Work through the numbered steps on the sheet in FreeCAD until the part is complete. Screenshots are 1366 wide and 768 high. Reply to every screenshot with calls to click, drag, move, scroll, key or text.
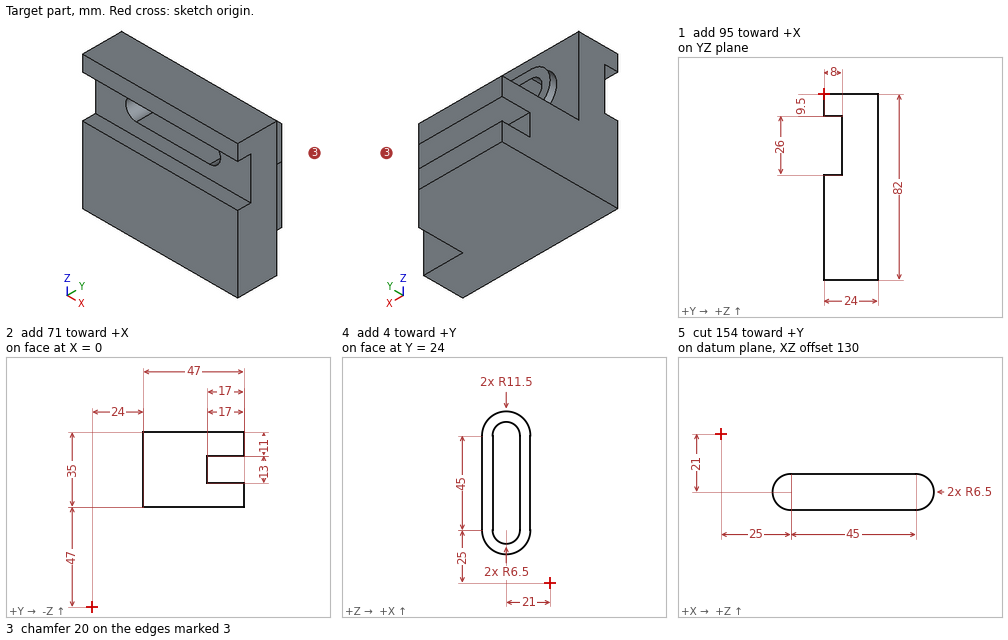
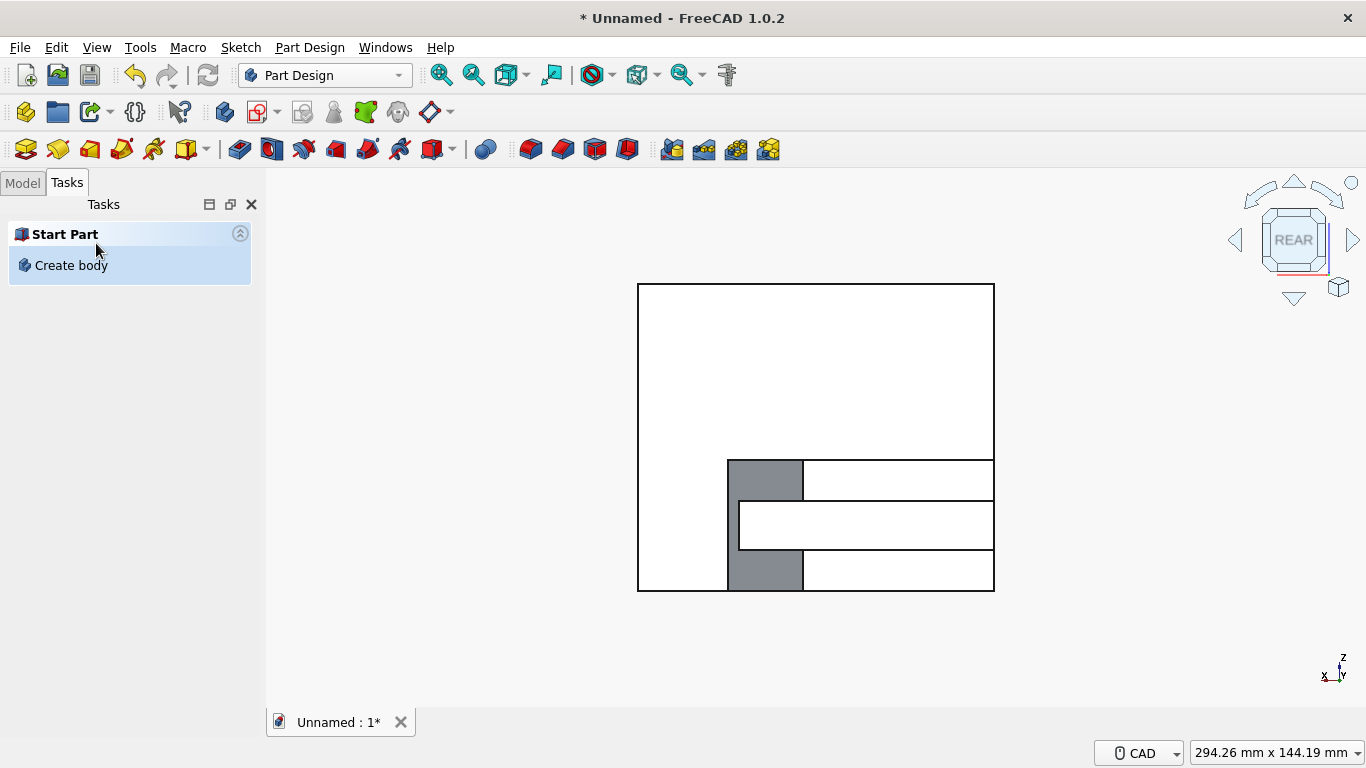
click(715, 393)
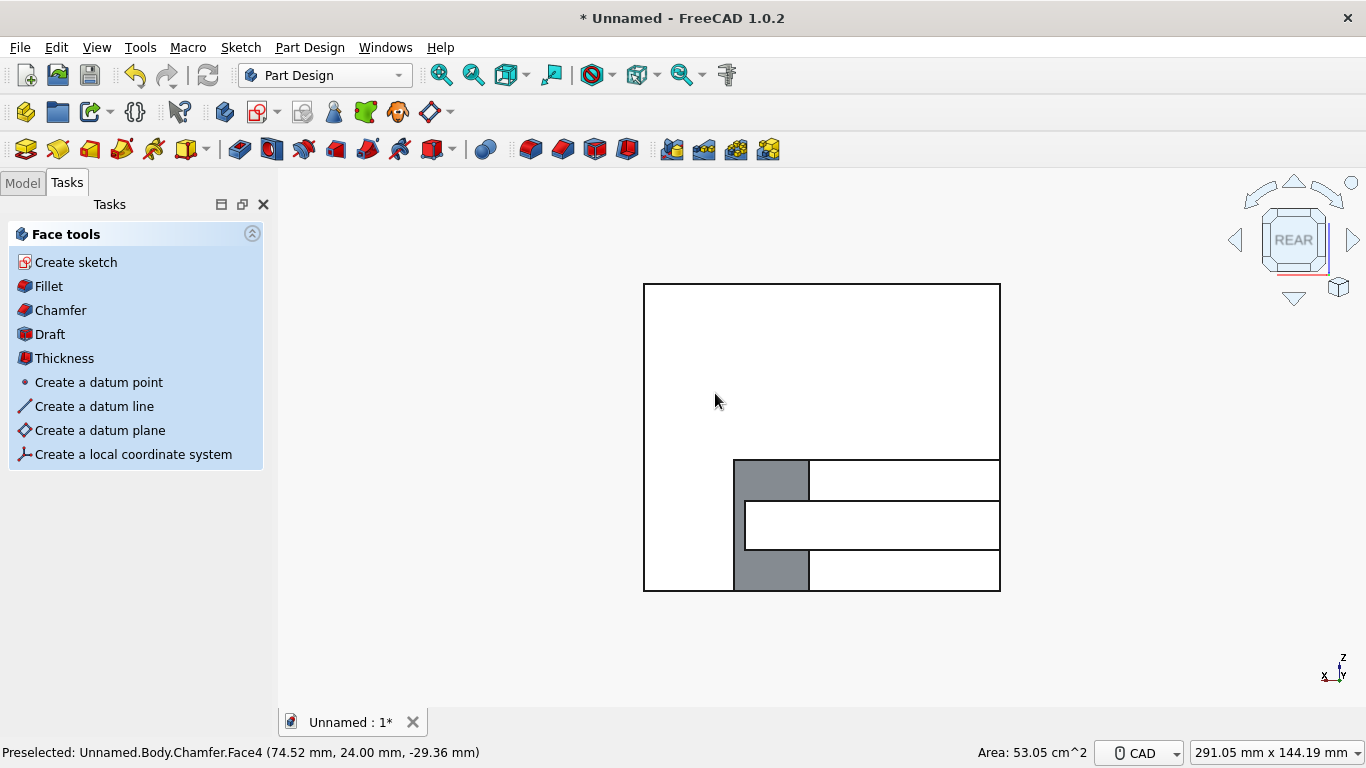
click(258, 112)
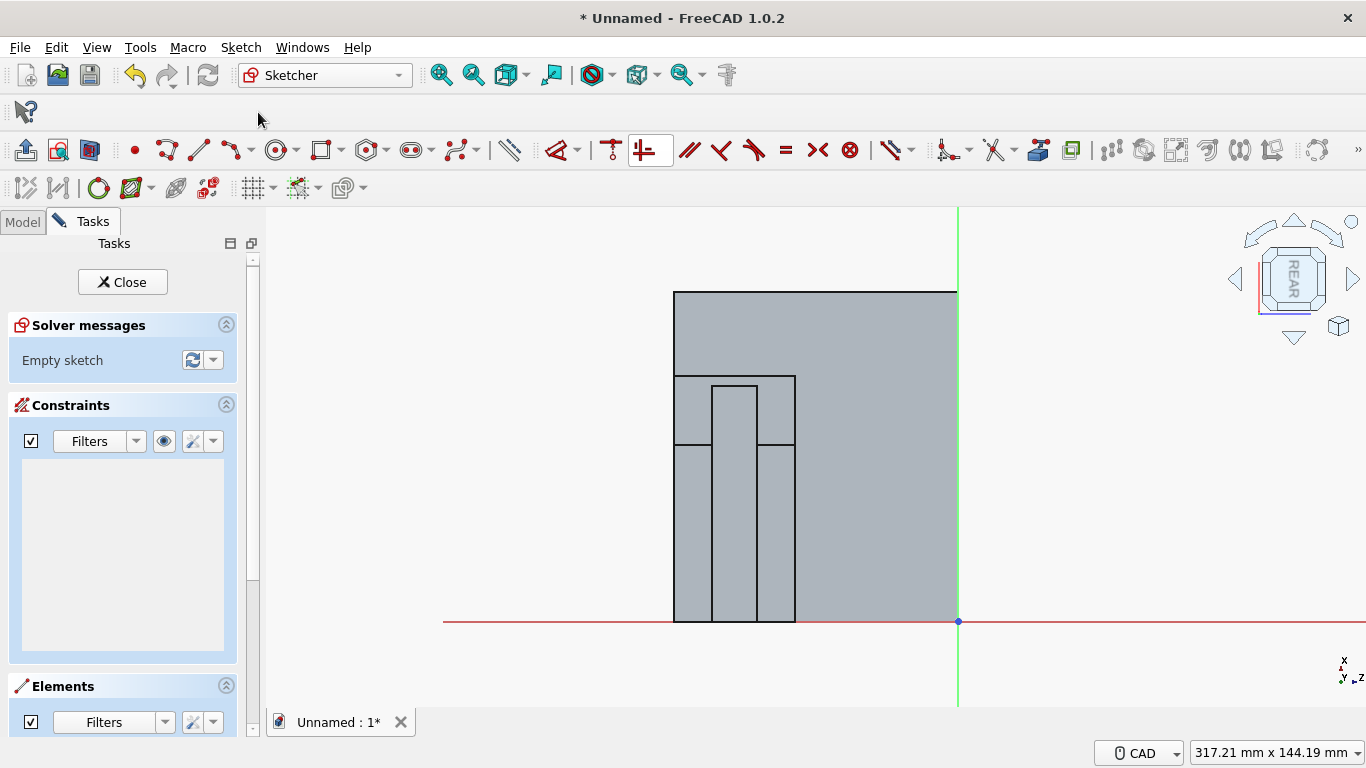
click(90, 150)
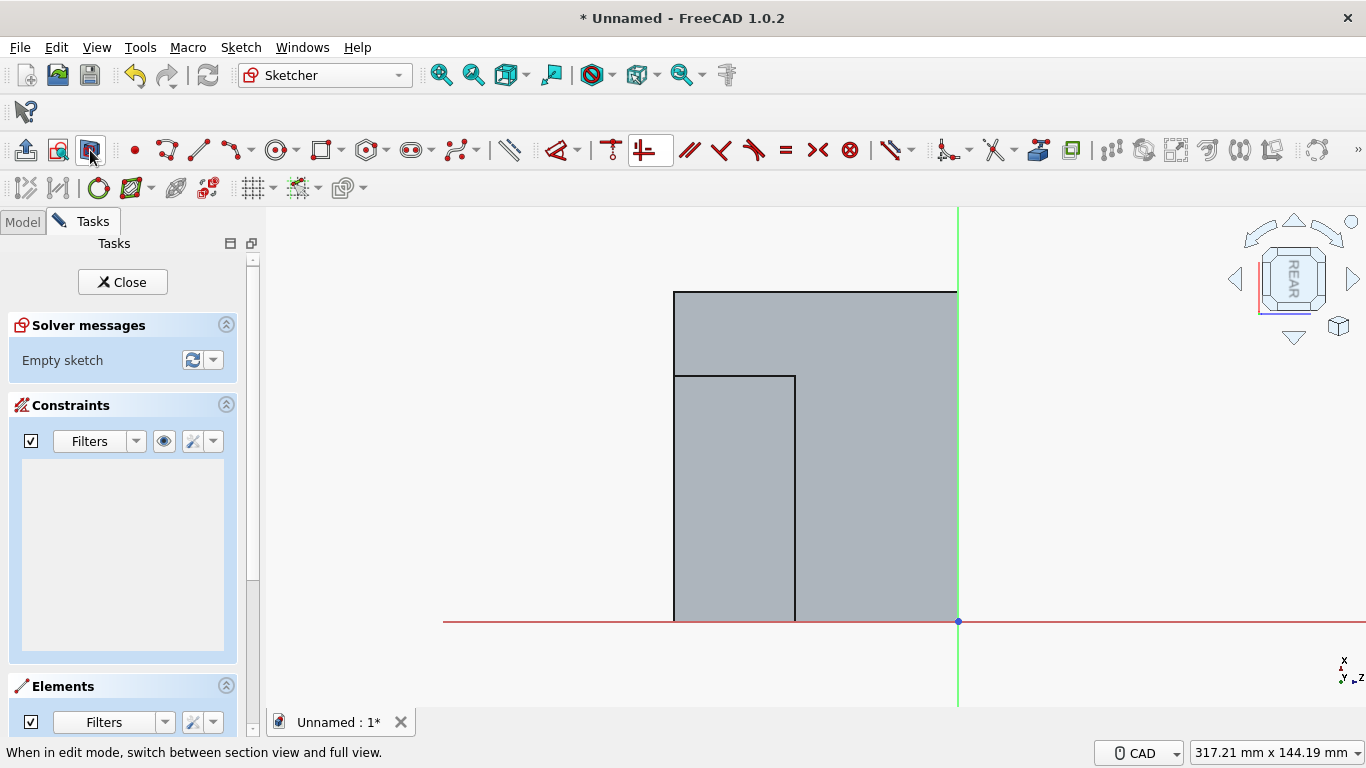
click(412, 150)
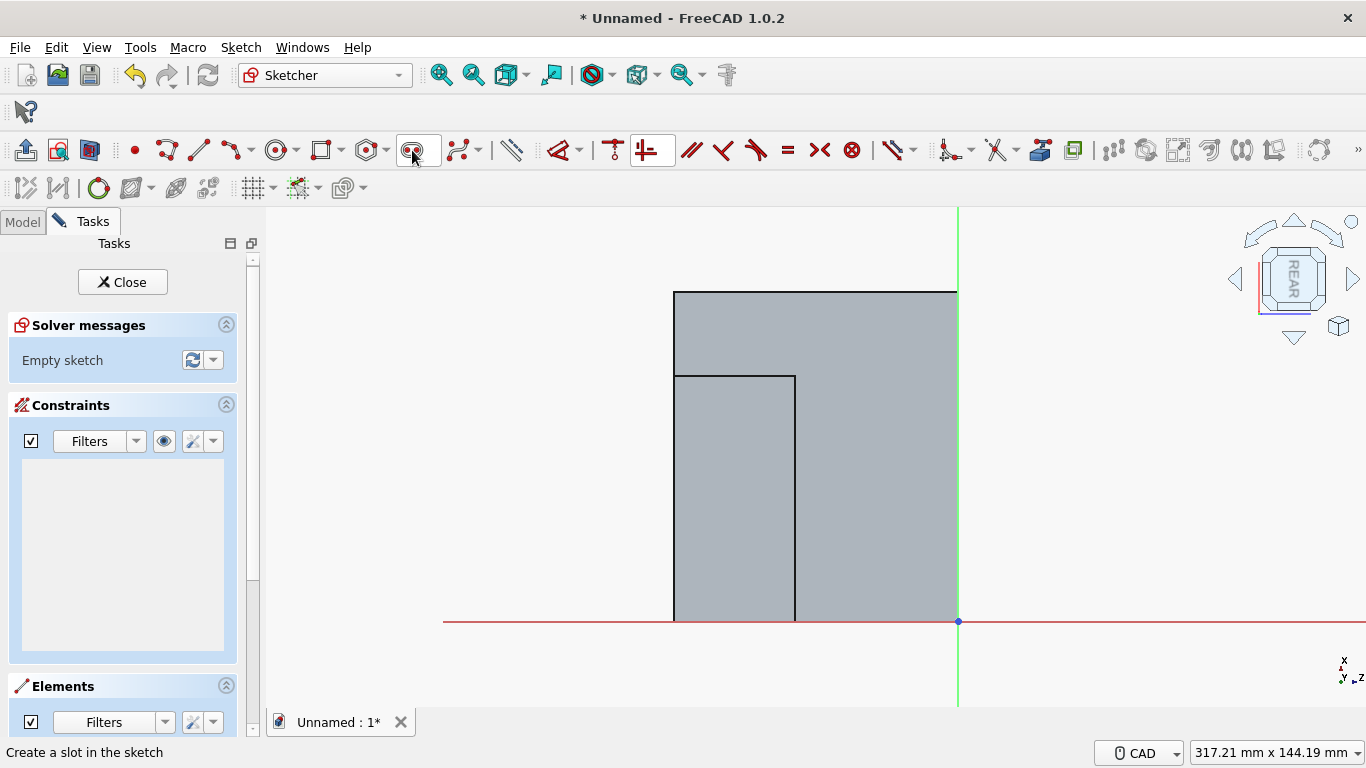
click(885, 535)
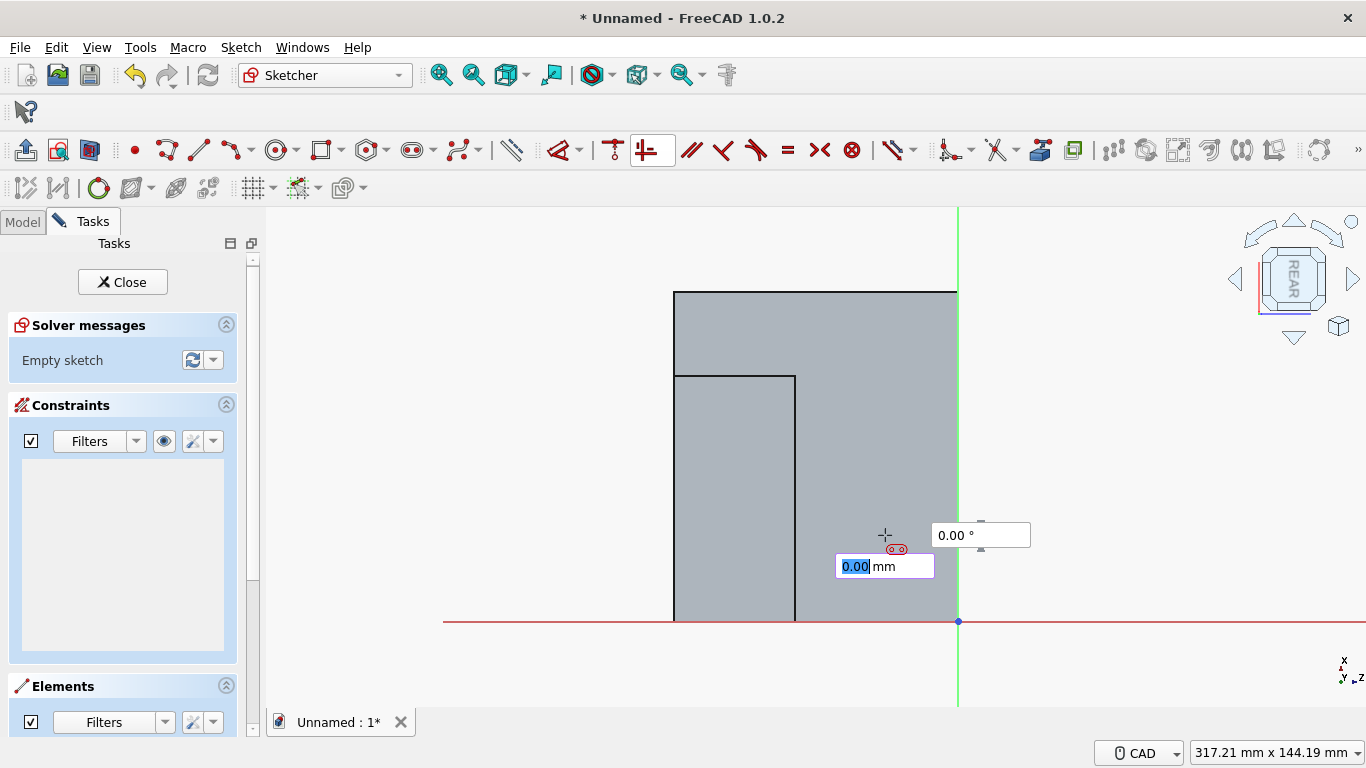
click(885, 379)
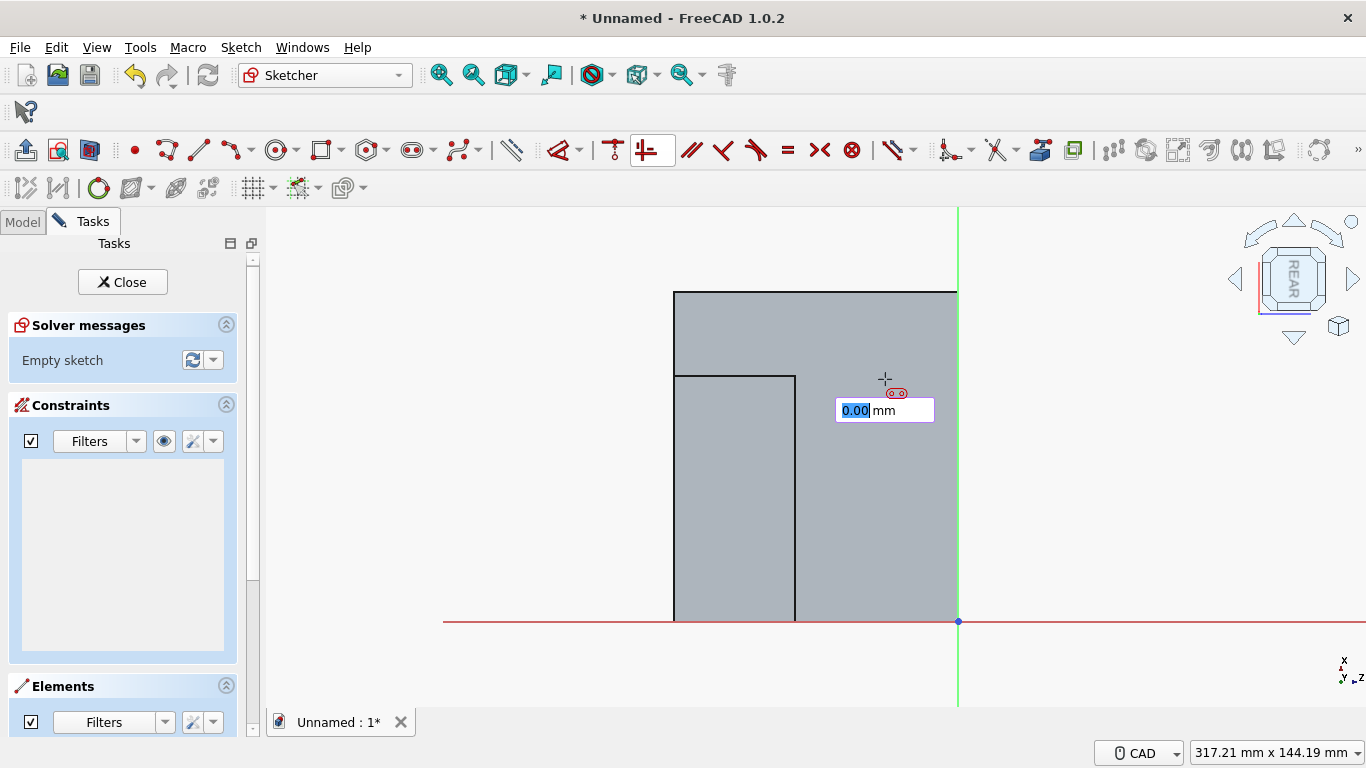
click(845, 457)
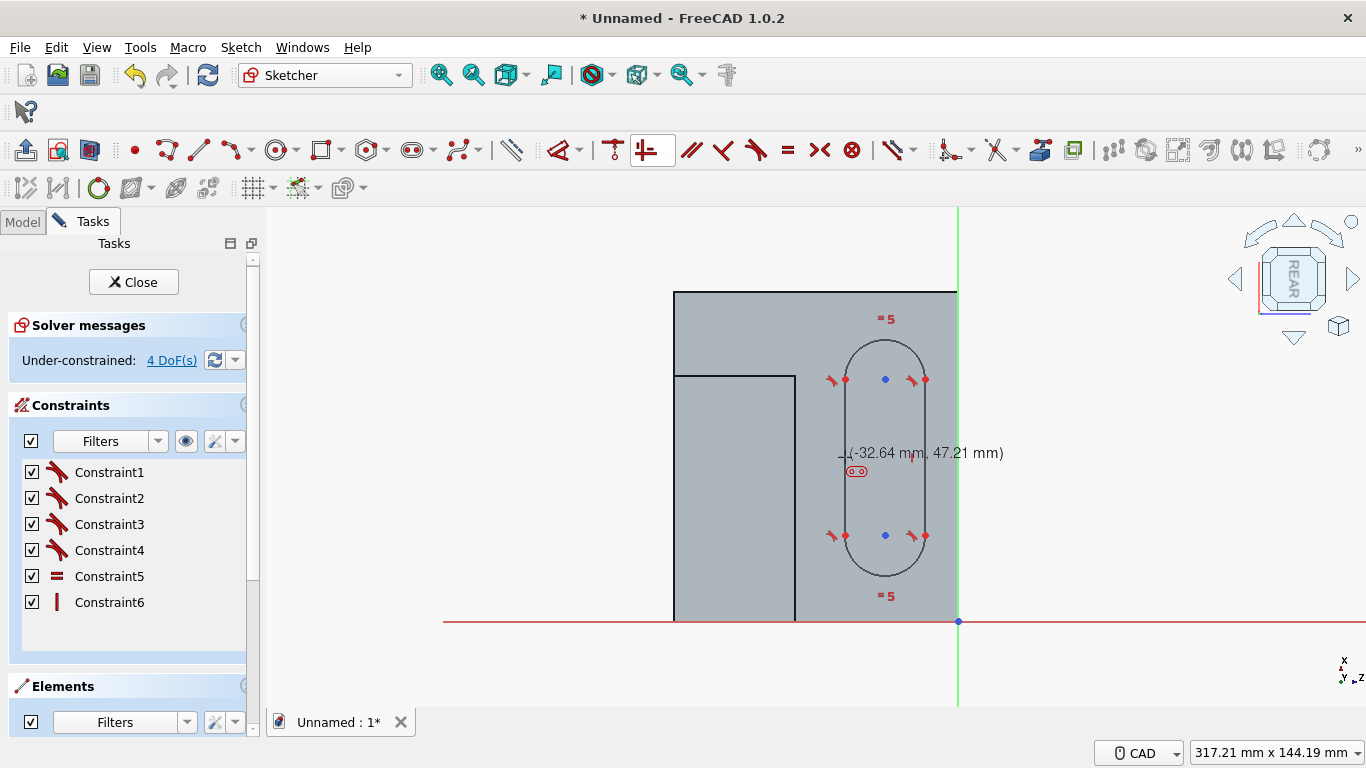
click(885, 536)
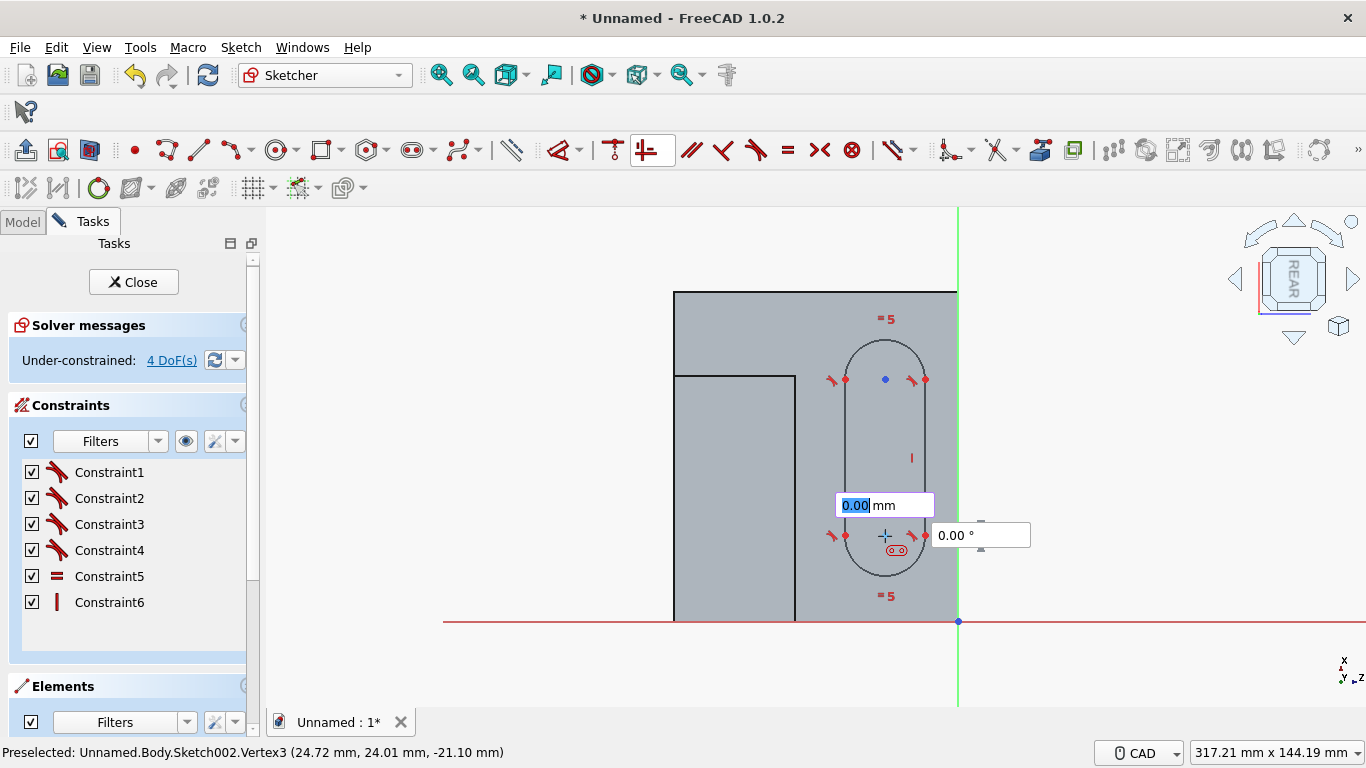
click(885, 380)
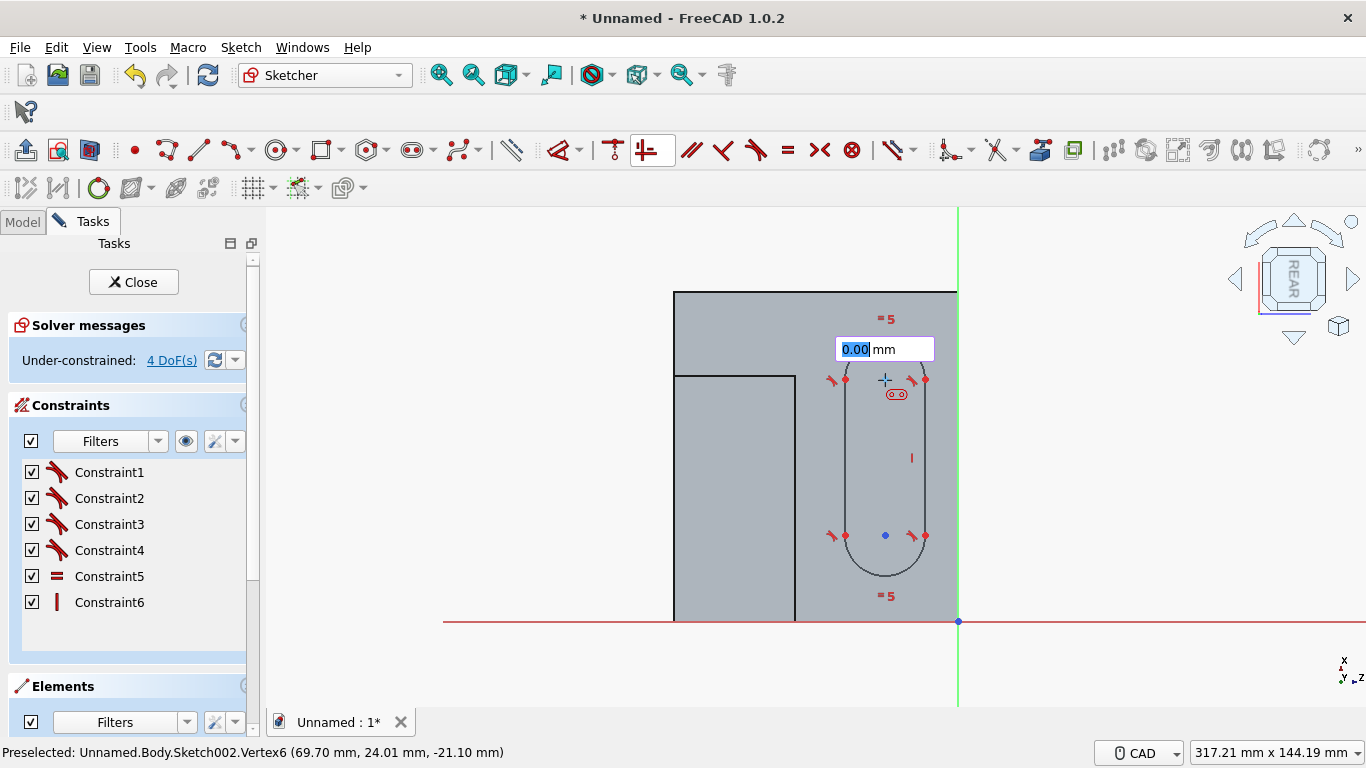
click(863, 457)
key(Escape)